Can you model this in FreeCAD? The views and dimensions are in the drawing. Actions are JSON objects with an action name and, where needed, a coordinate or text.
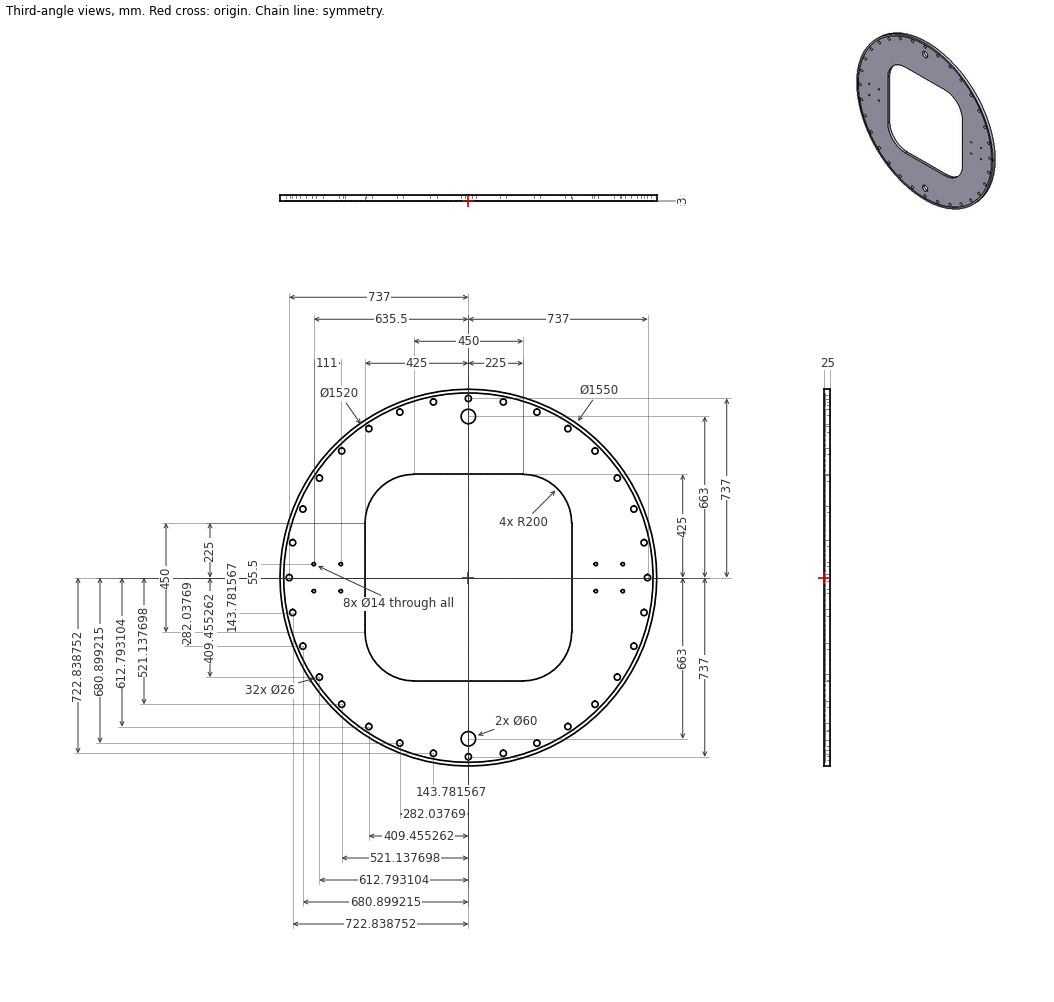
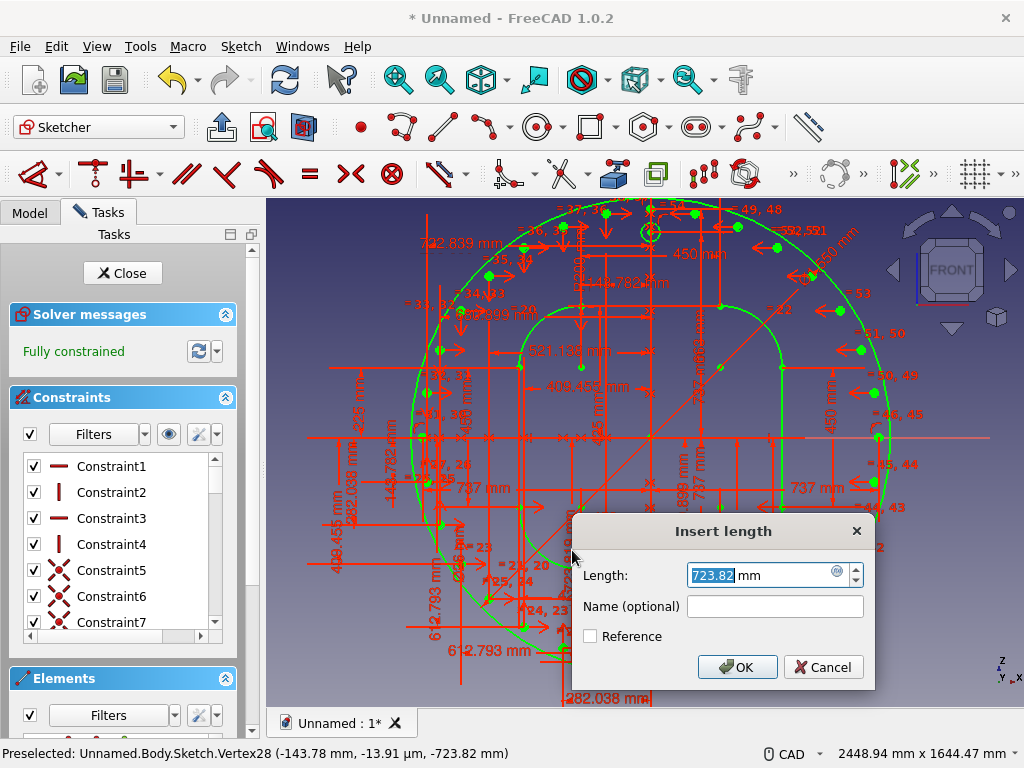
{"action": "type", "text": "722.838752"}
{"action": "key", "text": "Return"}
{"action": "key", "text": "Escape"}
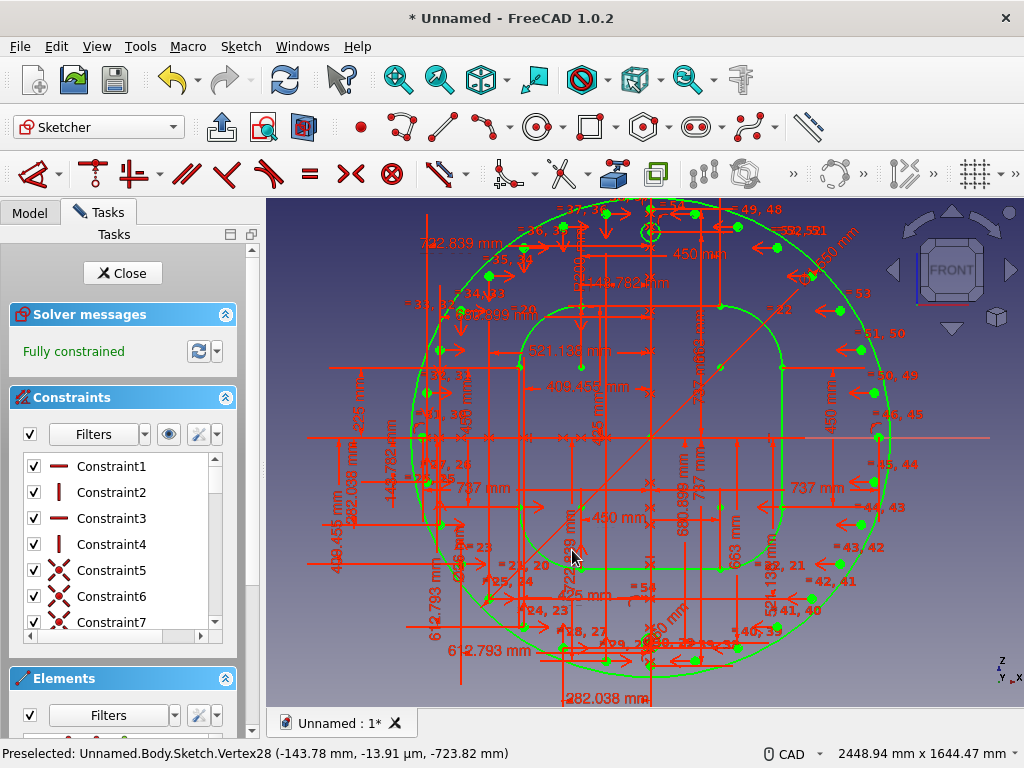
{"action": "left_click", "coordinate": [123, 273]}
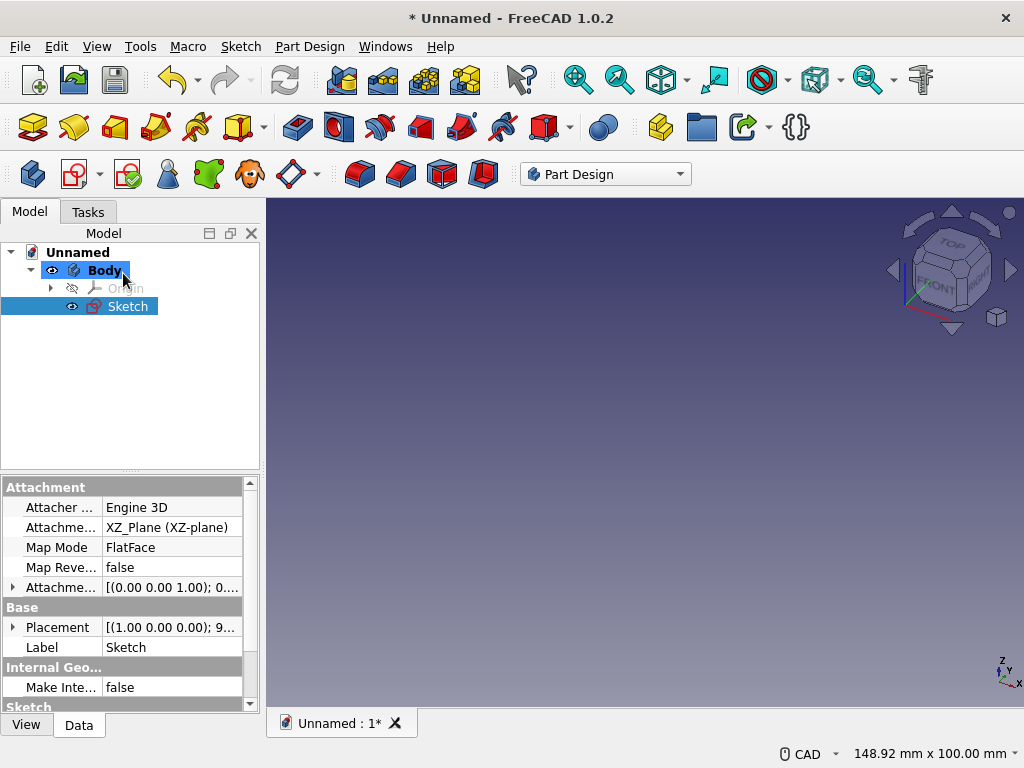
{"action": "left_click", "coordinate": [33, 128]}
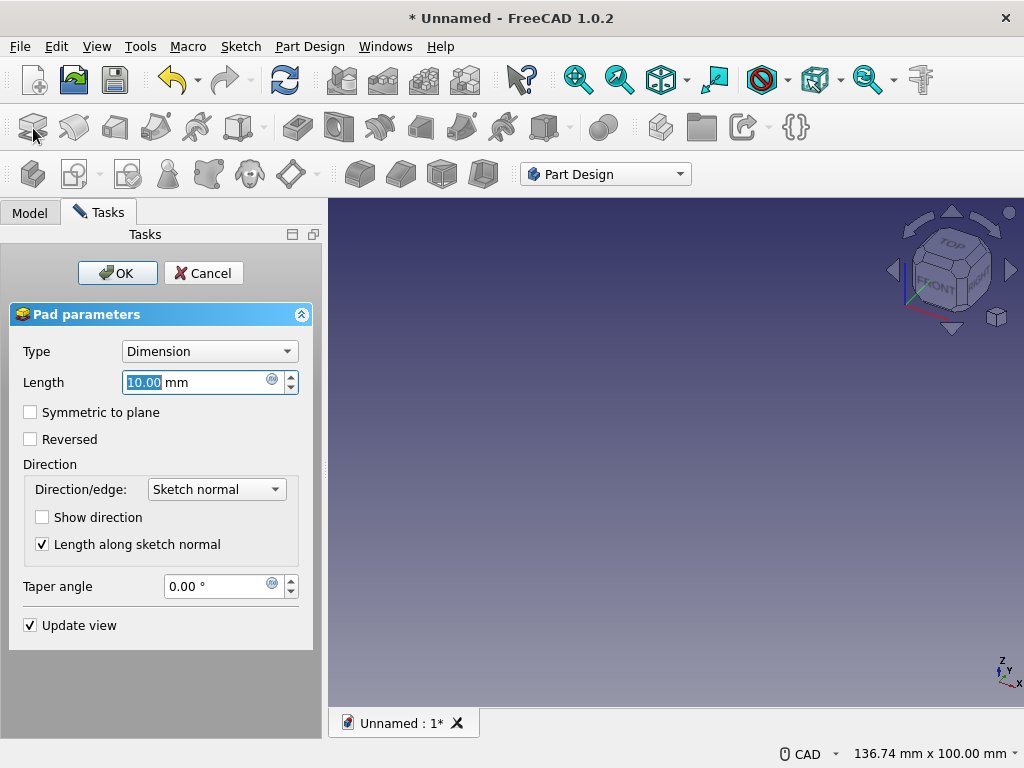
{"action": "type", "text": "25"}
{"action": "key", "text": "Tab"}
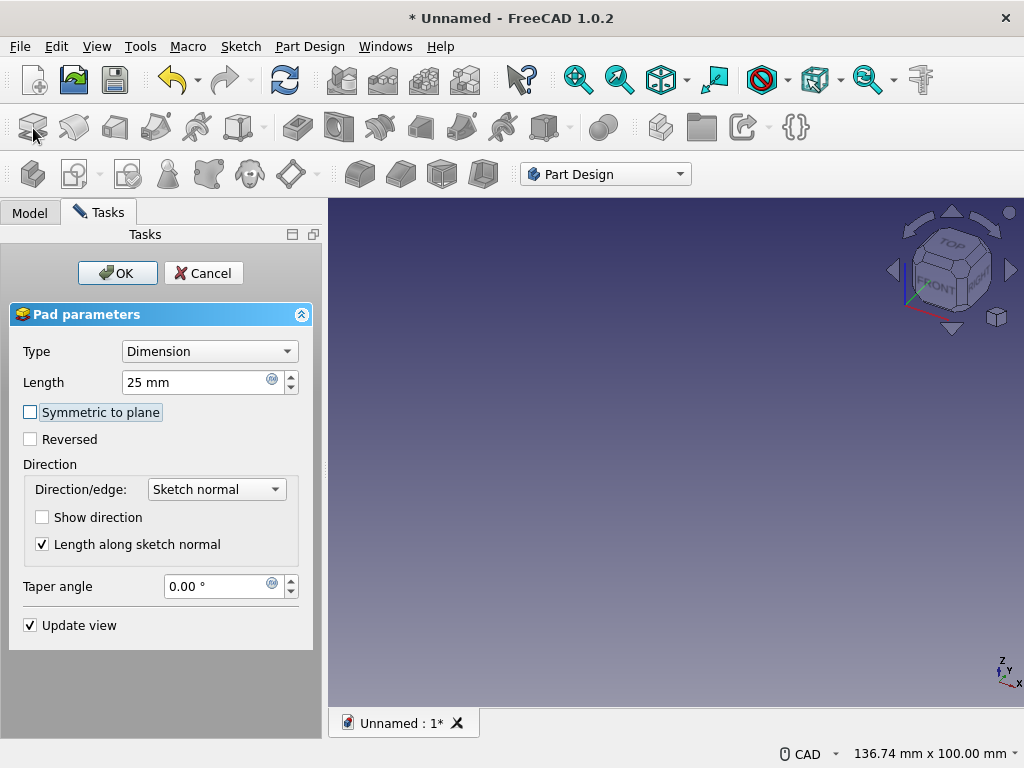
{"action": "left_click", "coordinate": [31, 439]}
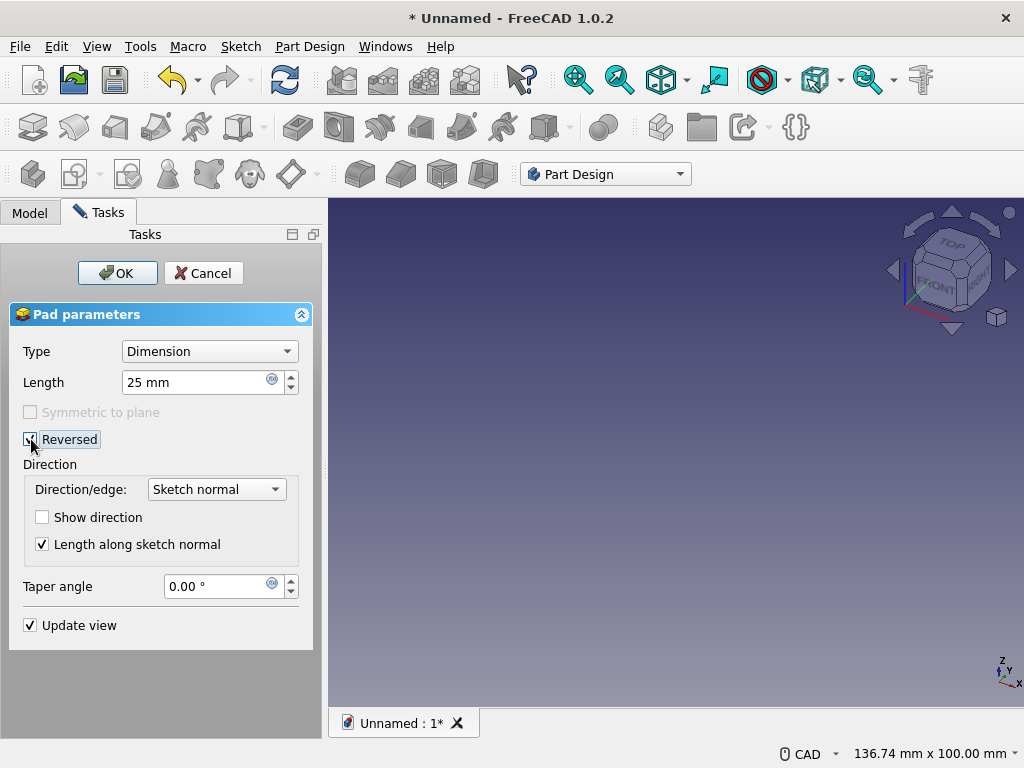
{"action": "left_click", "coordinate": [118, 273]}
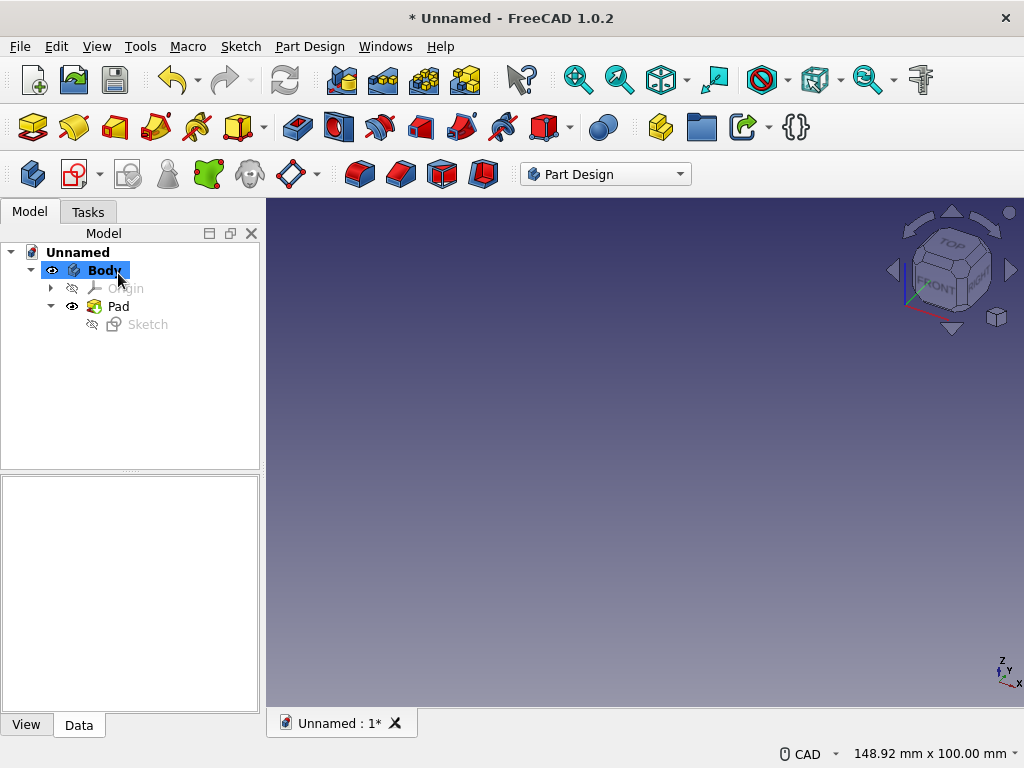
{"action": "left_click", "coordinate": [579, 80]}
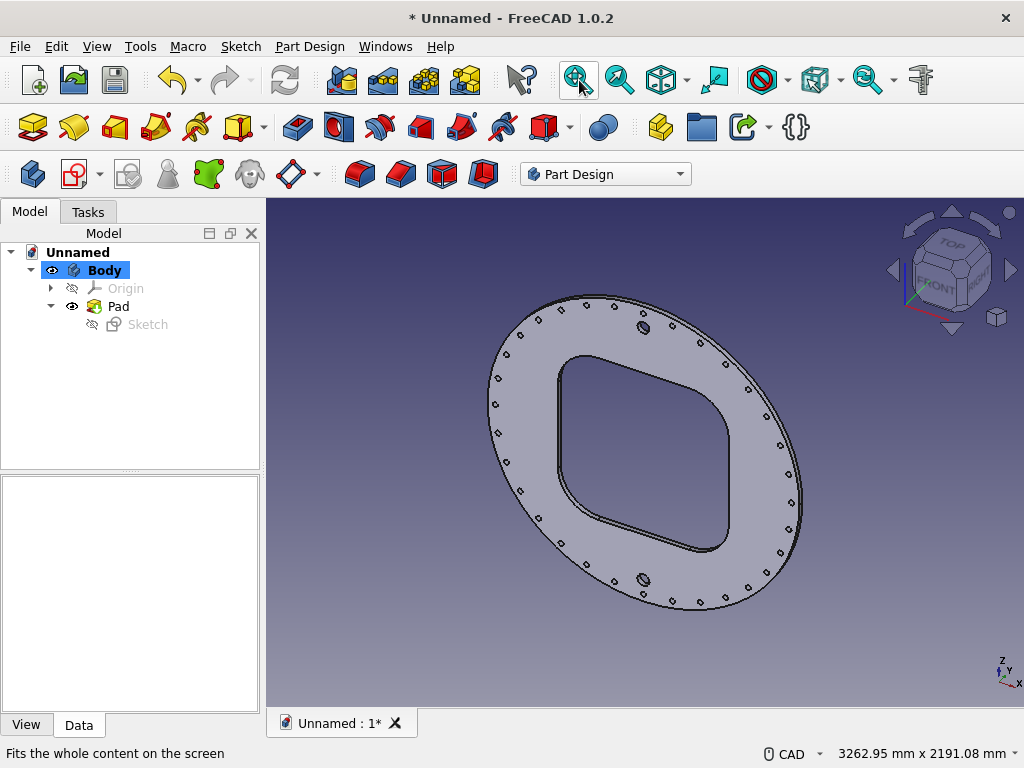
{"action": "key", "text": "4"}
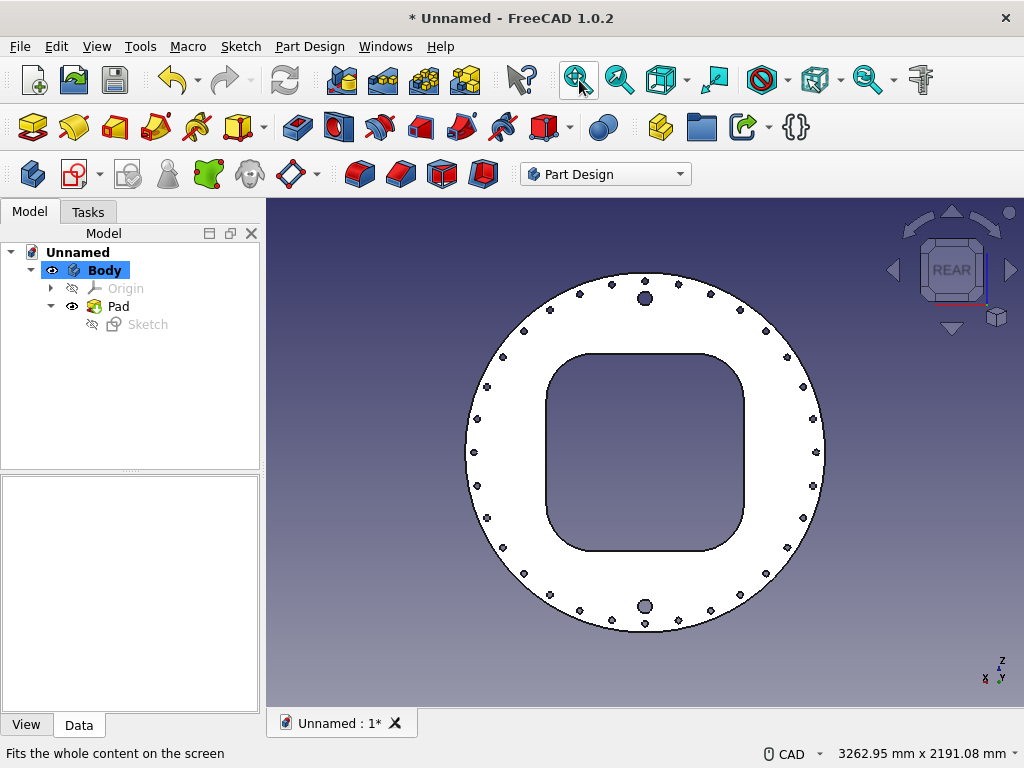
{"action": "left_click", "coordinate": [542, 554]}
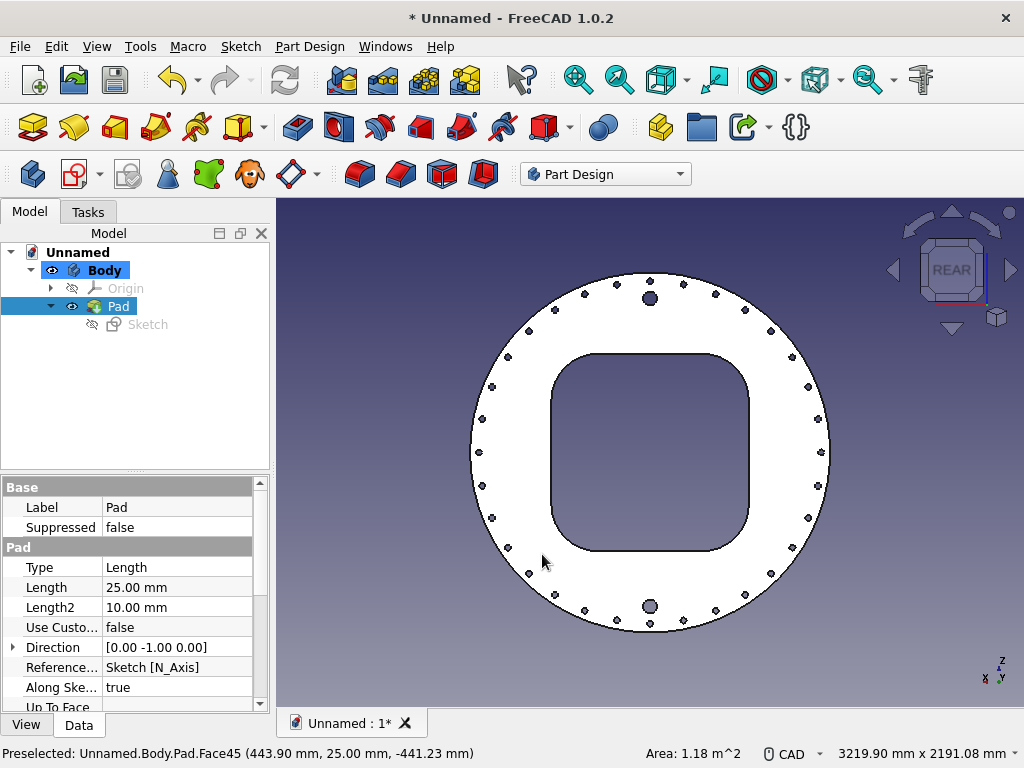
{"action": "left_click", "coordinate": [74, 174]}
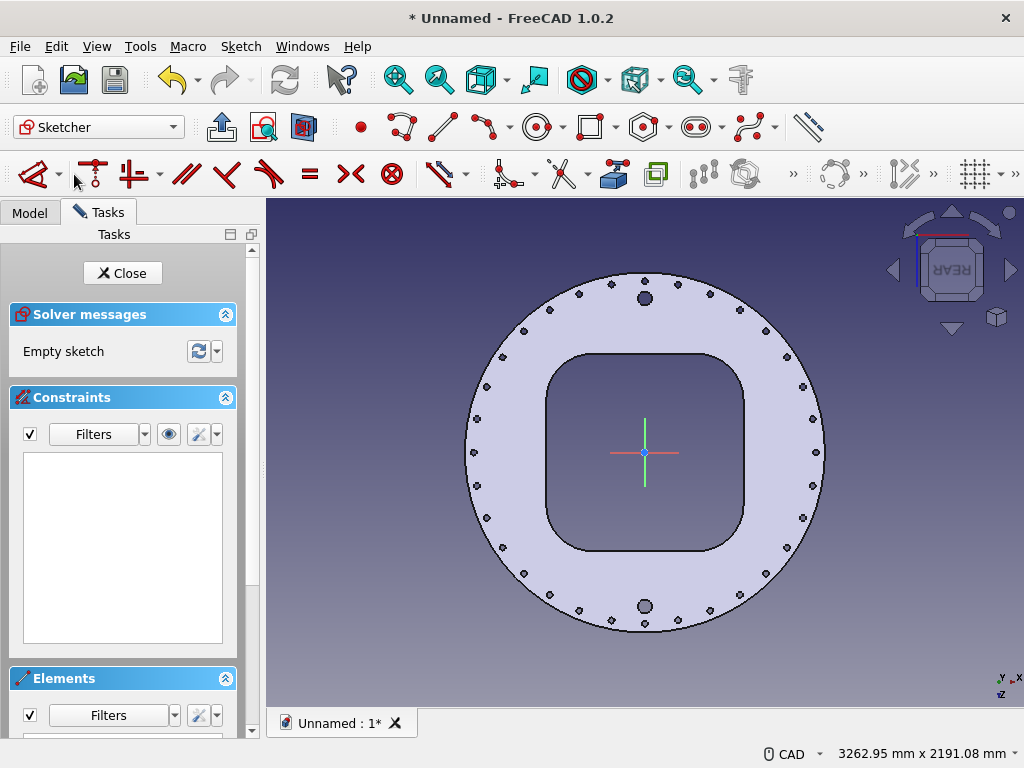
{"action": "left_click", "coordinate": [536, 128]}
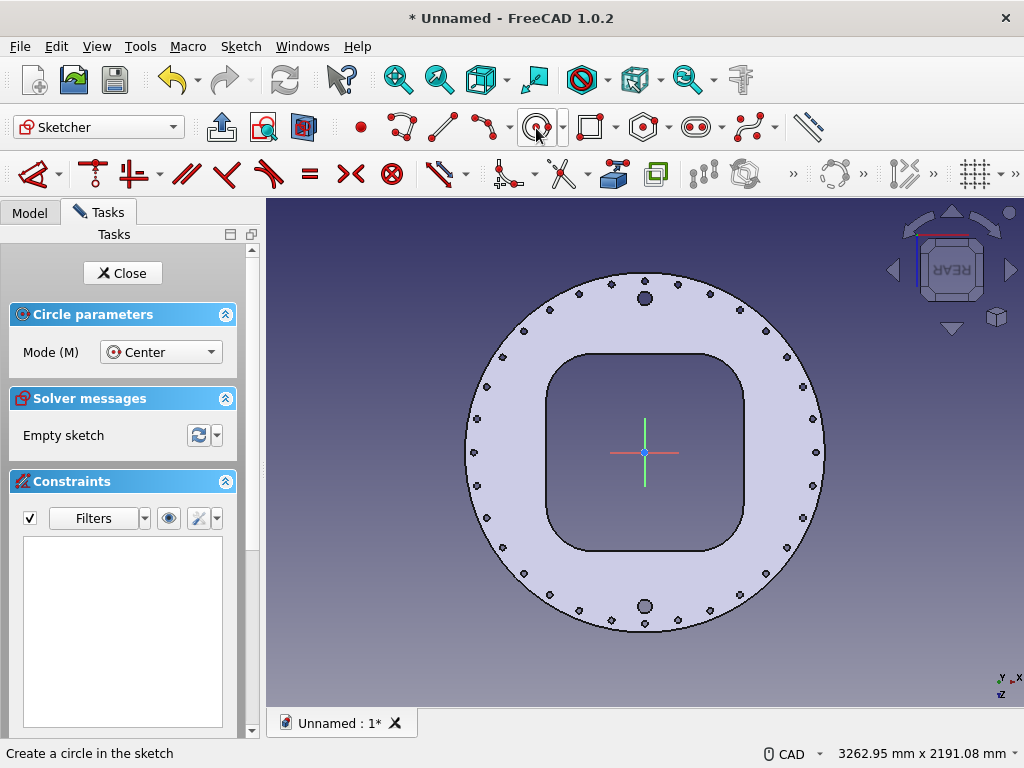
{"action": "scroll", "coordinate": [497, 465], "scroll_direction": "up", "scroll_amount": 14}